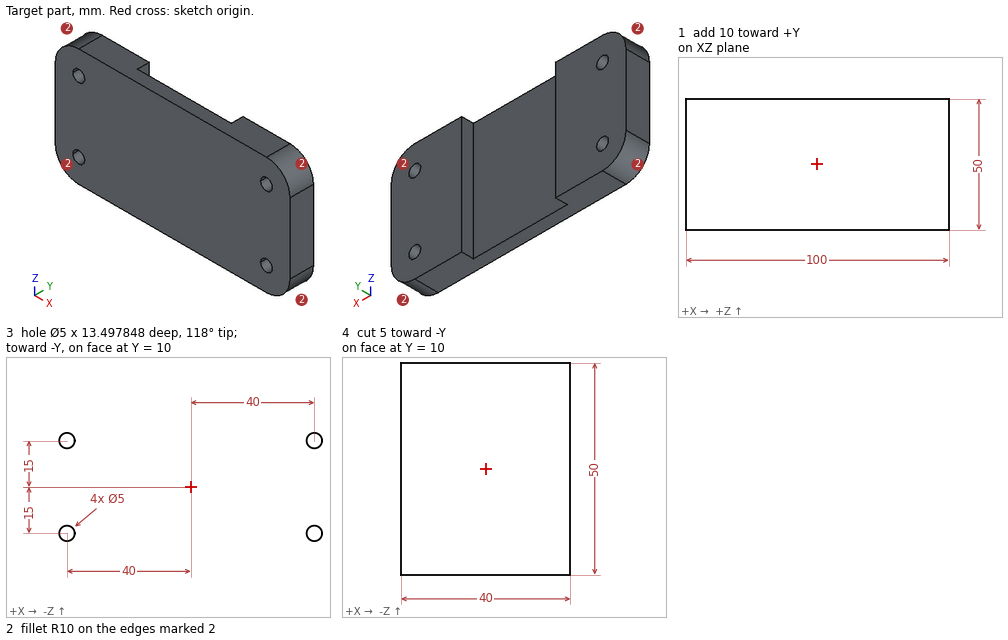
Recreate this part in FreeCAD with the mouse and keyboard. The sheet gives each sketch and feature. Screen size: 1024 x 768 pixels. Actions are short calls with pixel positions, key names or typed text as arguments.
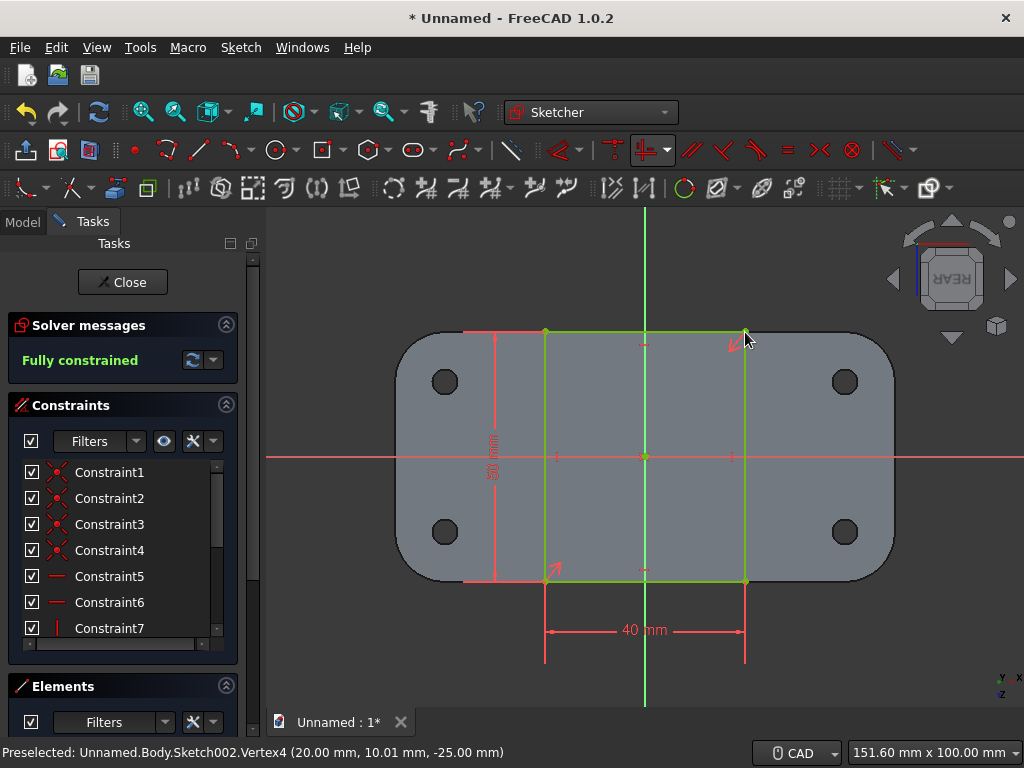
click(123, 282)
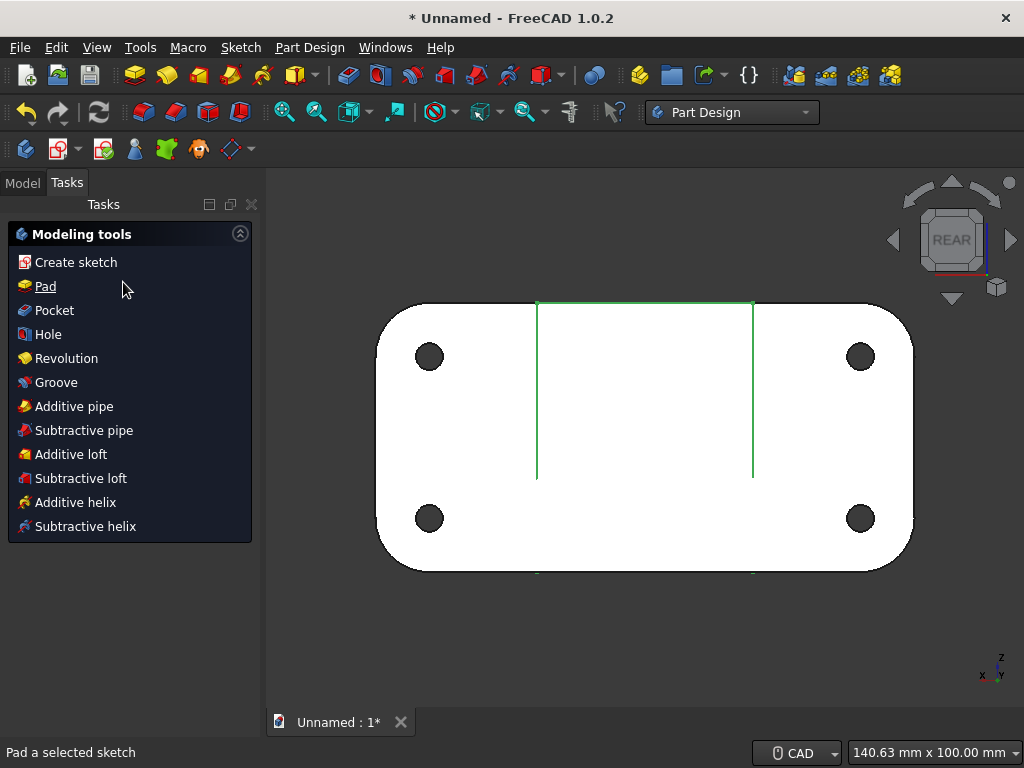
click(350, 76)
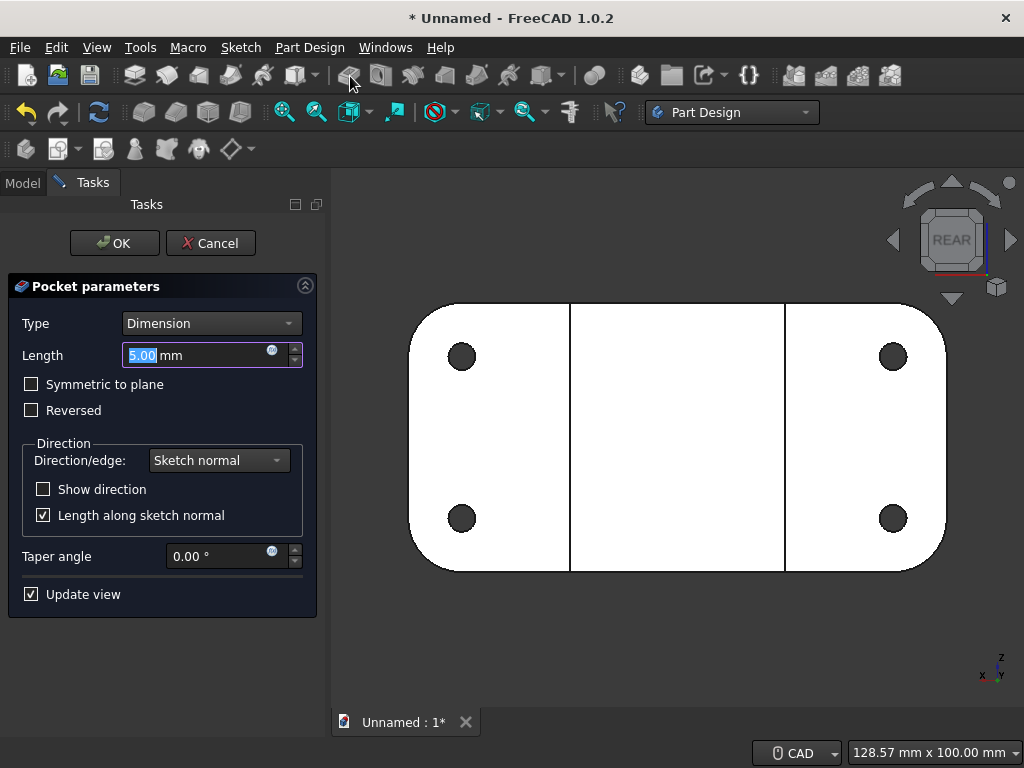
text(5)
key(Tab)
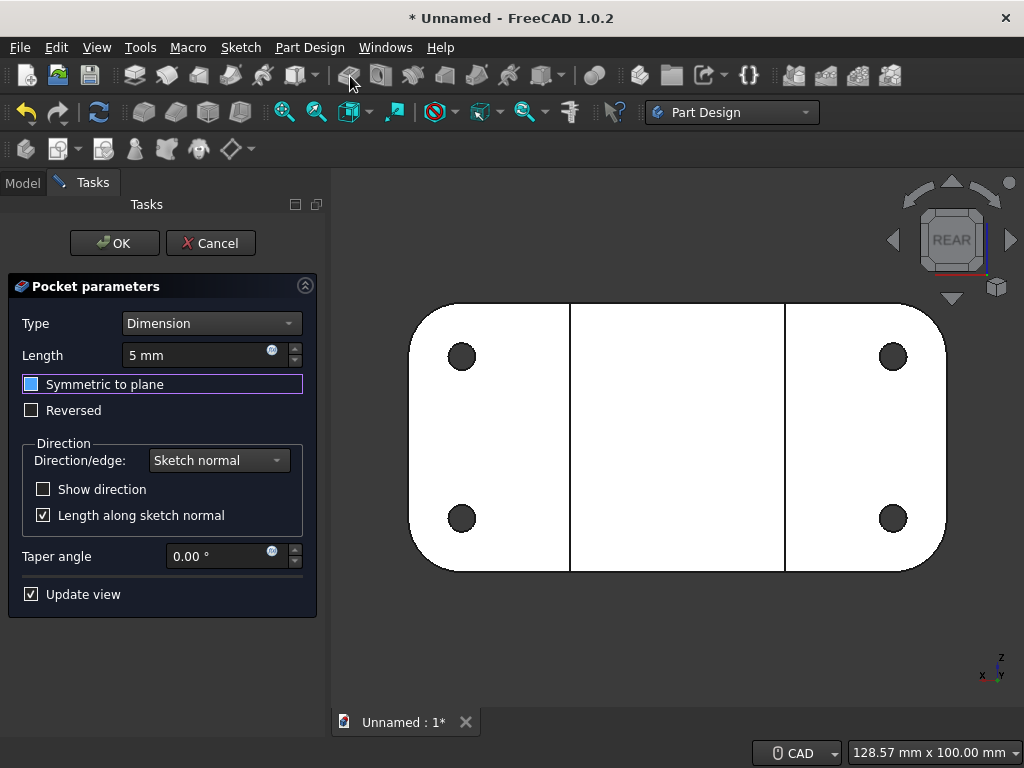
click(115, 243)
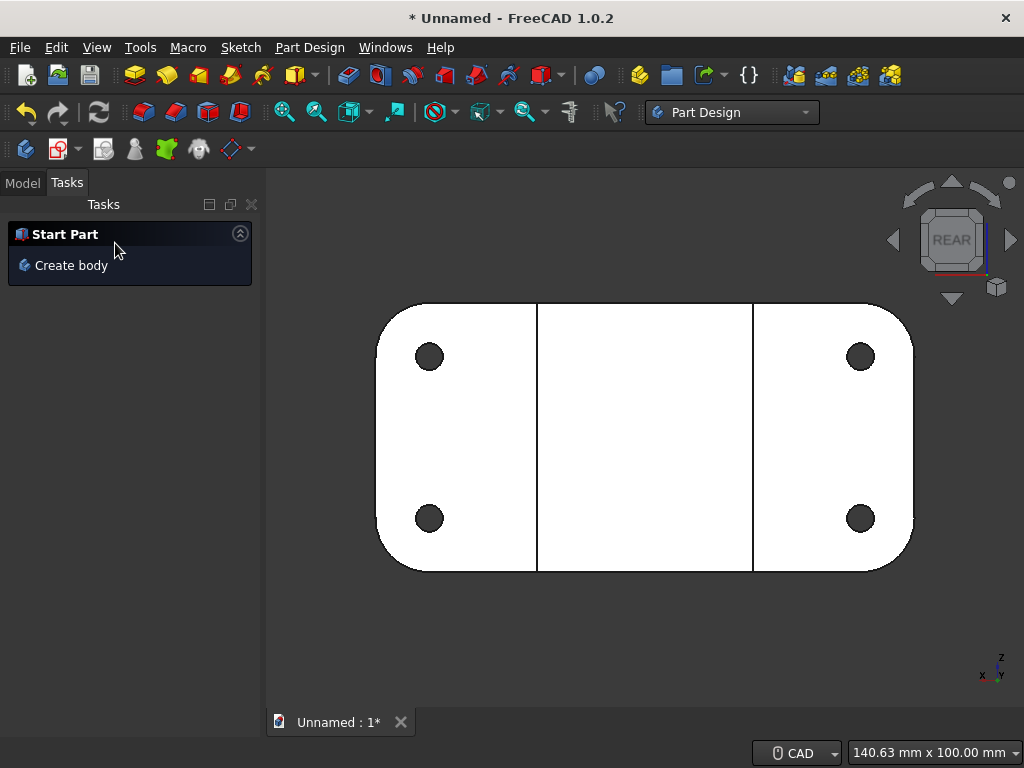
key(0)